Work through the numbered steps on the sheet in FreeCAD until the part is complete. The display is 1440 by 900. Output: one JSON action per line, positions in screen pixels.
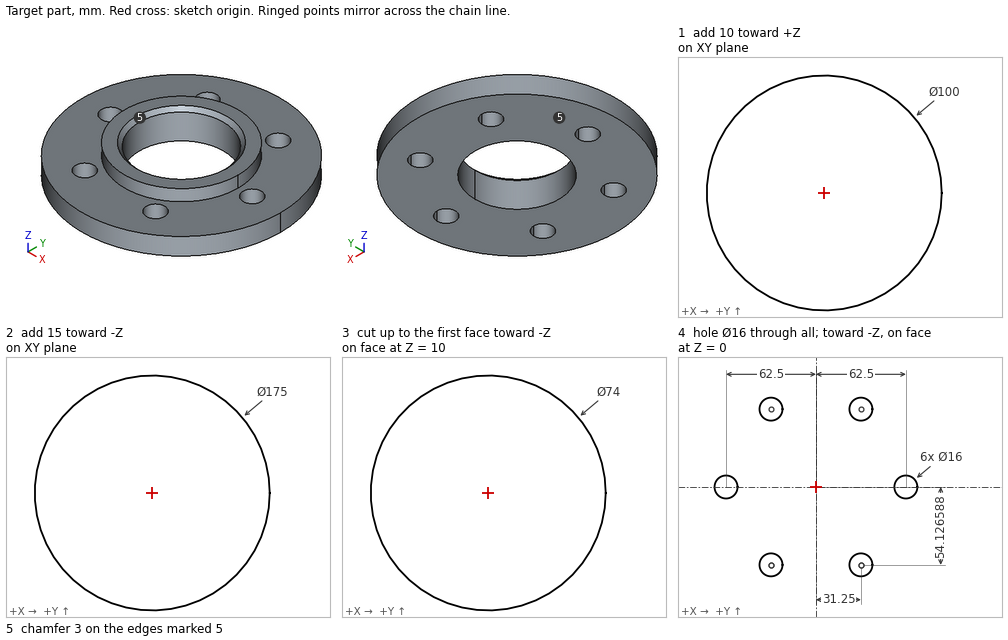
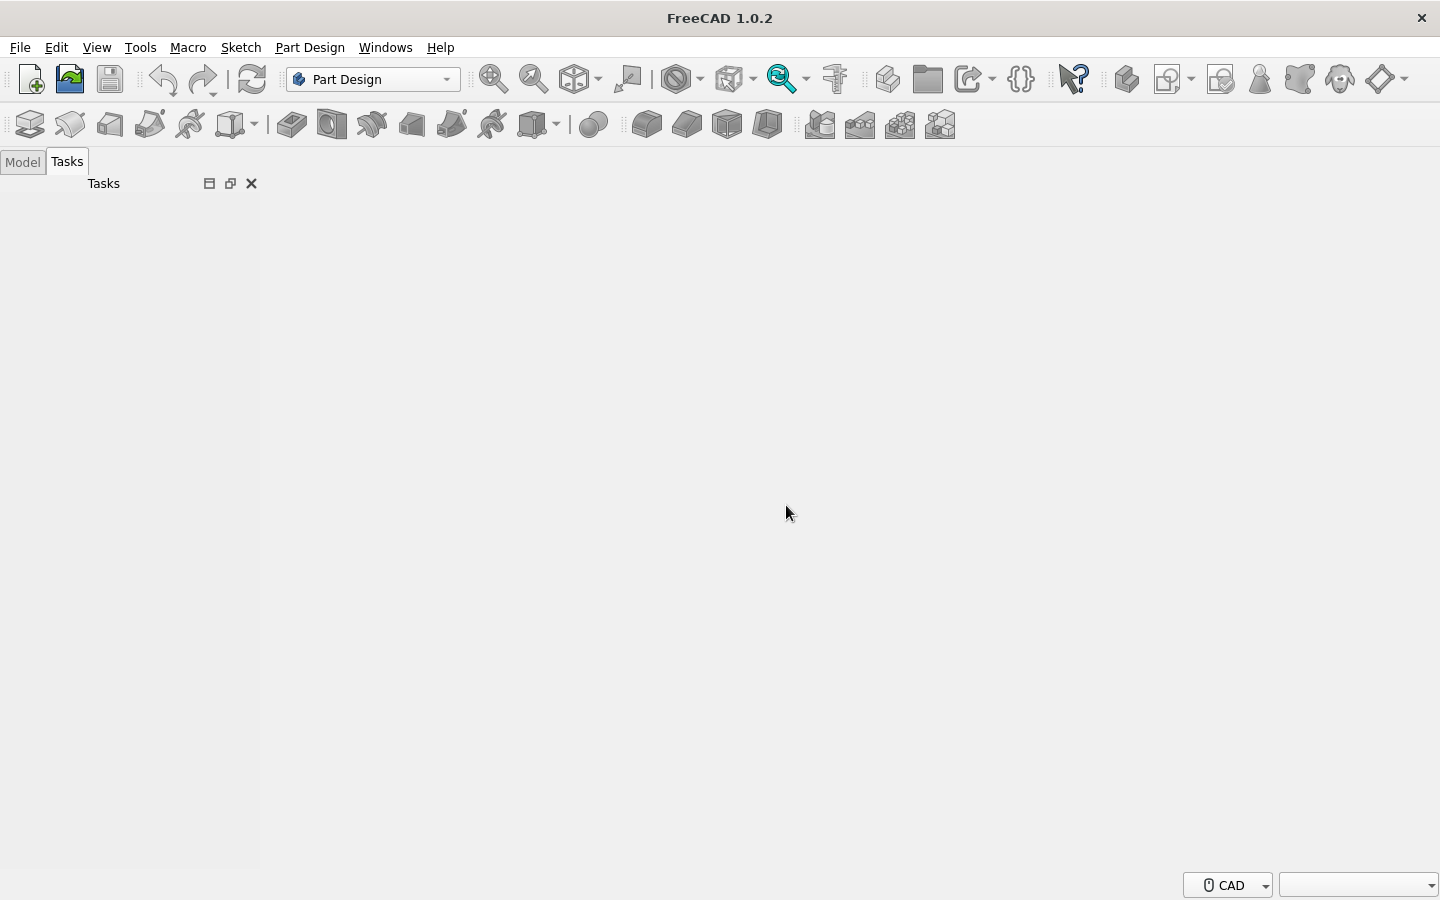
{"action": "left_click", "coordinate": [30, 80]}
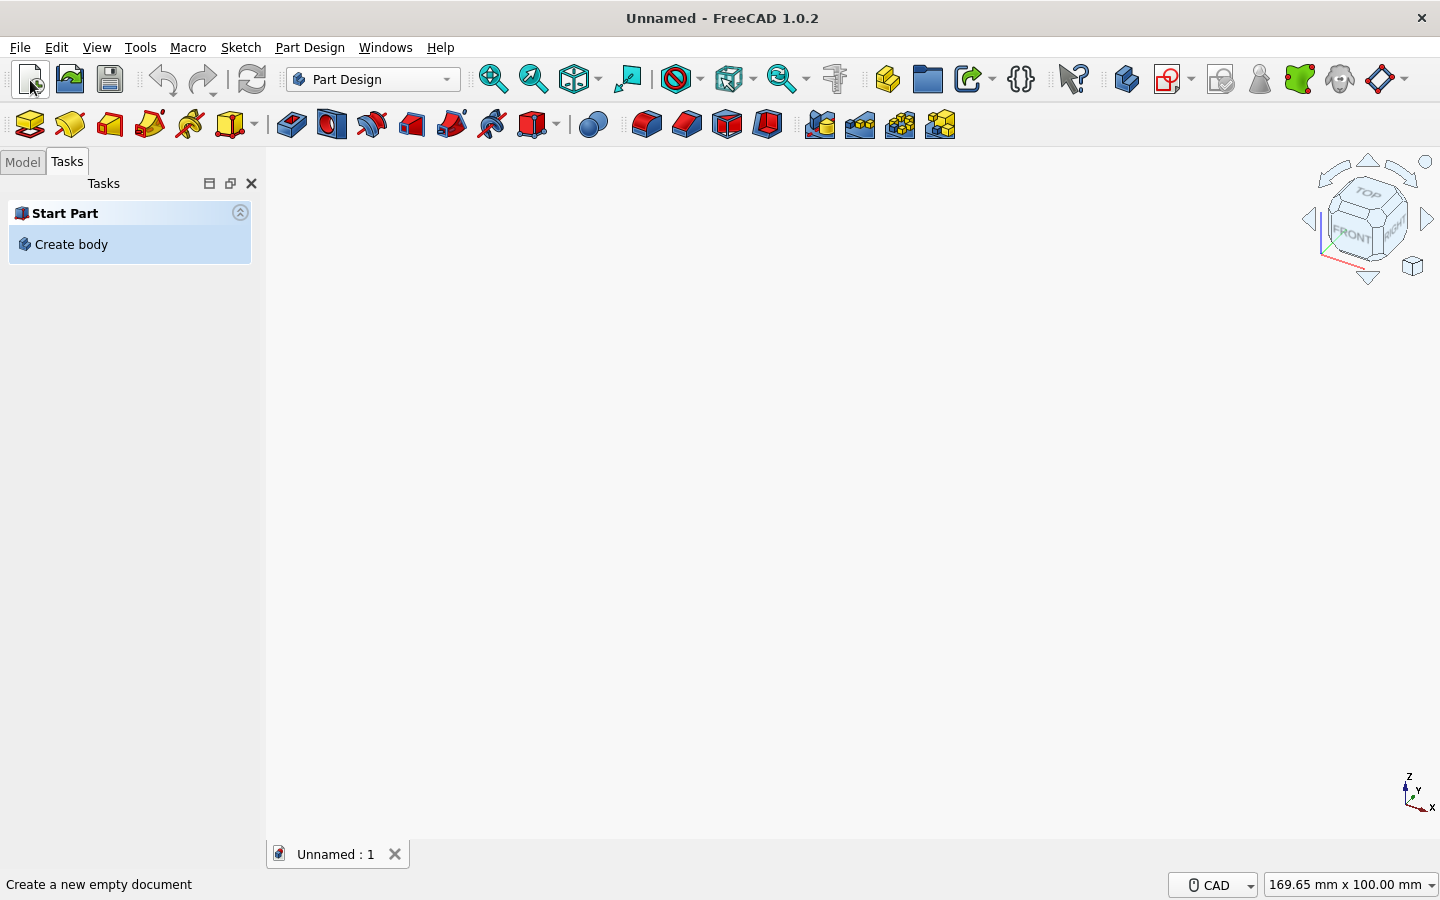
{"action": "left_click", "coordinate": [1168, 80]}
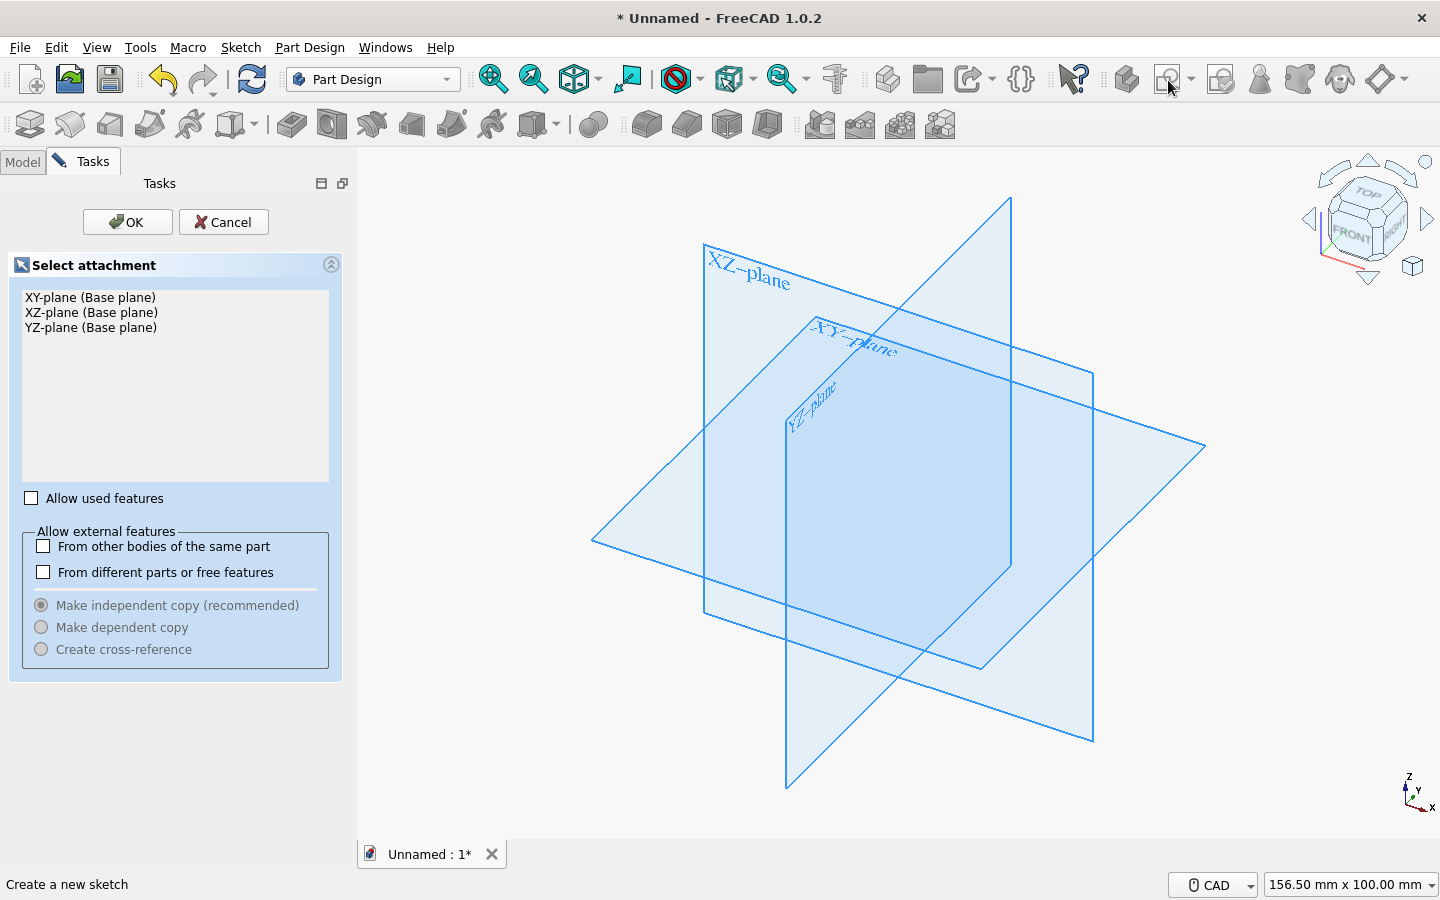
{"action": "left_click", "coordinate": [82, 298]}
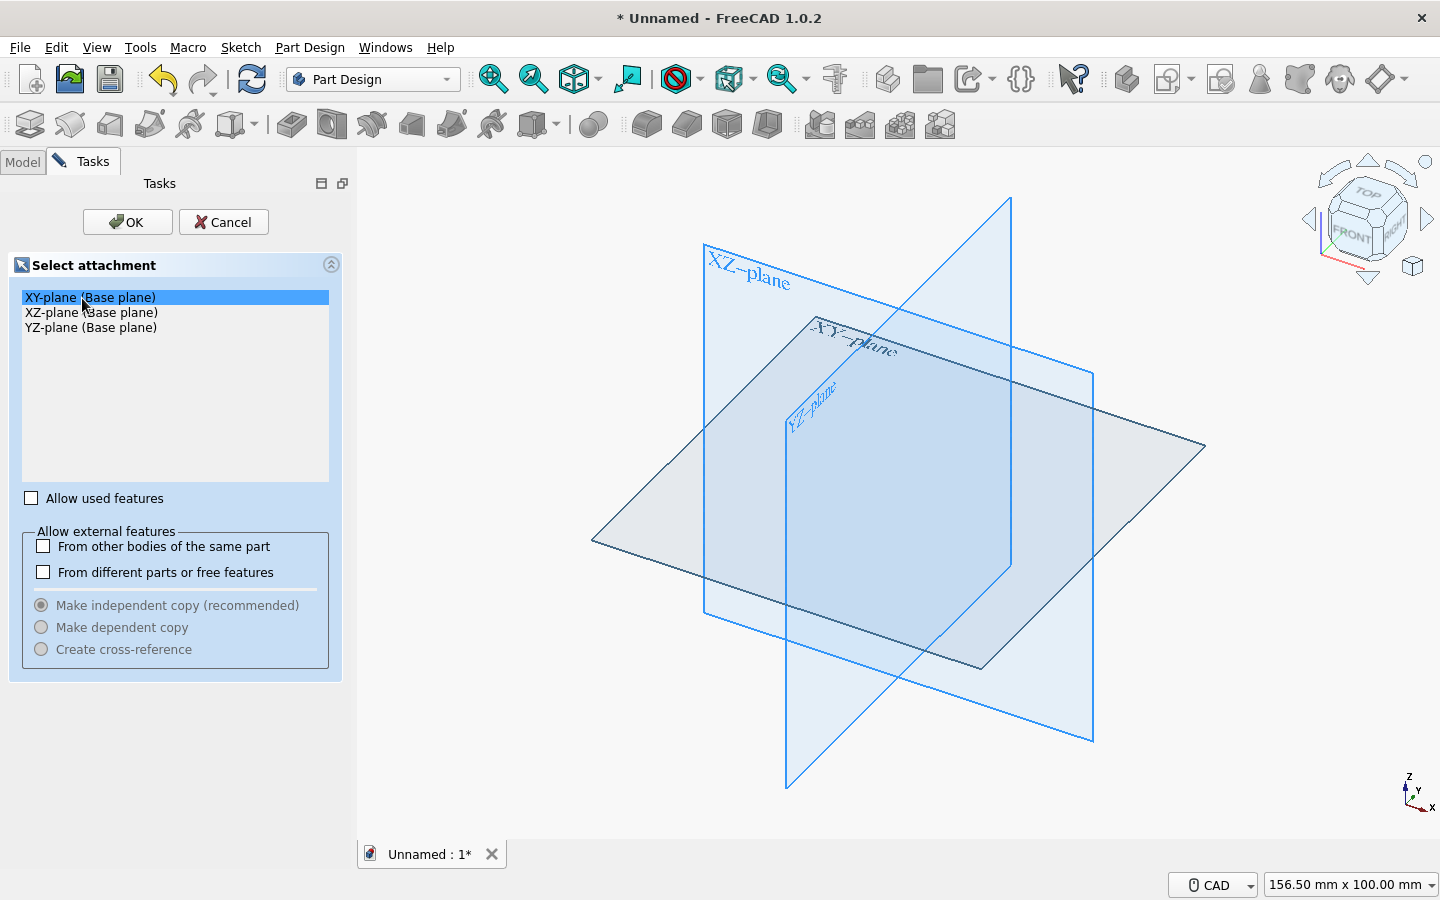
{"action": "left_click", "coordinate": [128, 222]}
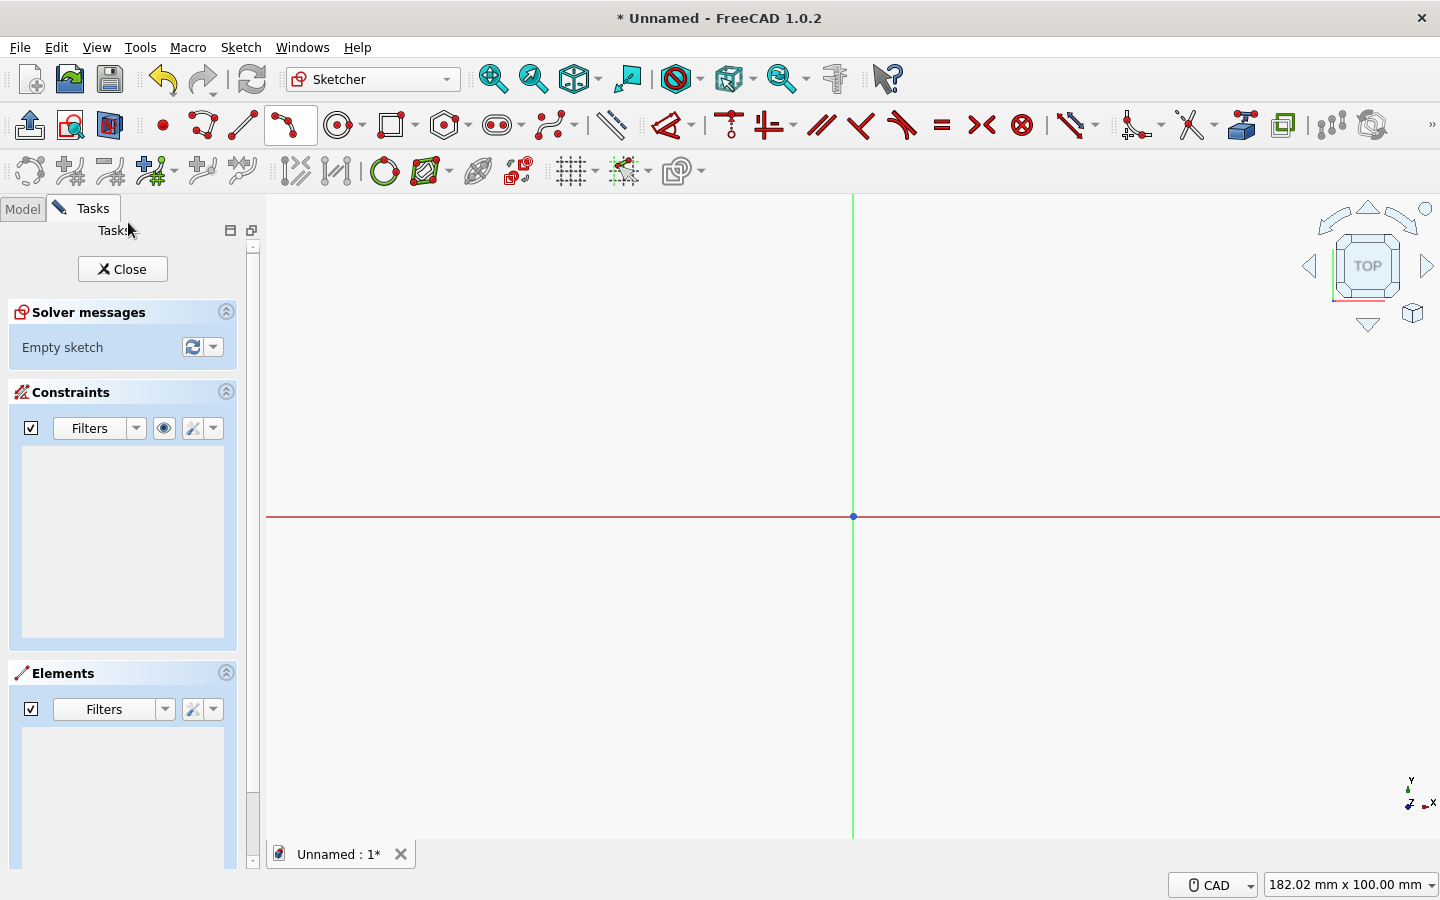
{"action": "scroll", "coordinate": [645, 516], "scroll_direction": "down", "scroll_amount": 2}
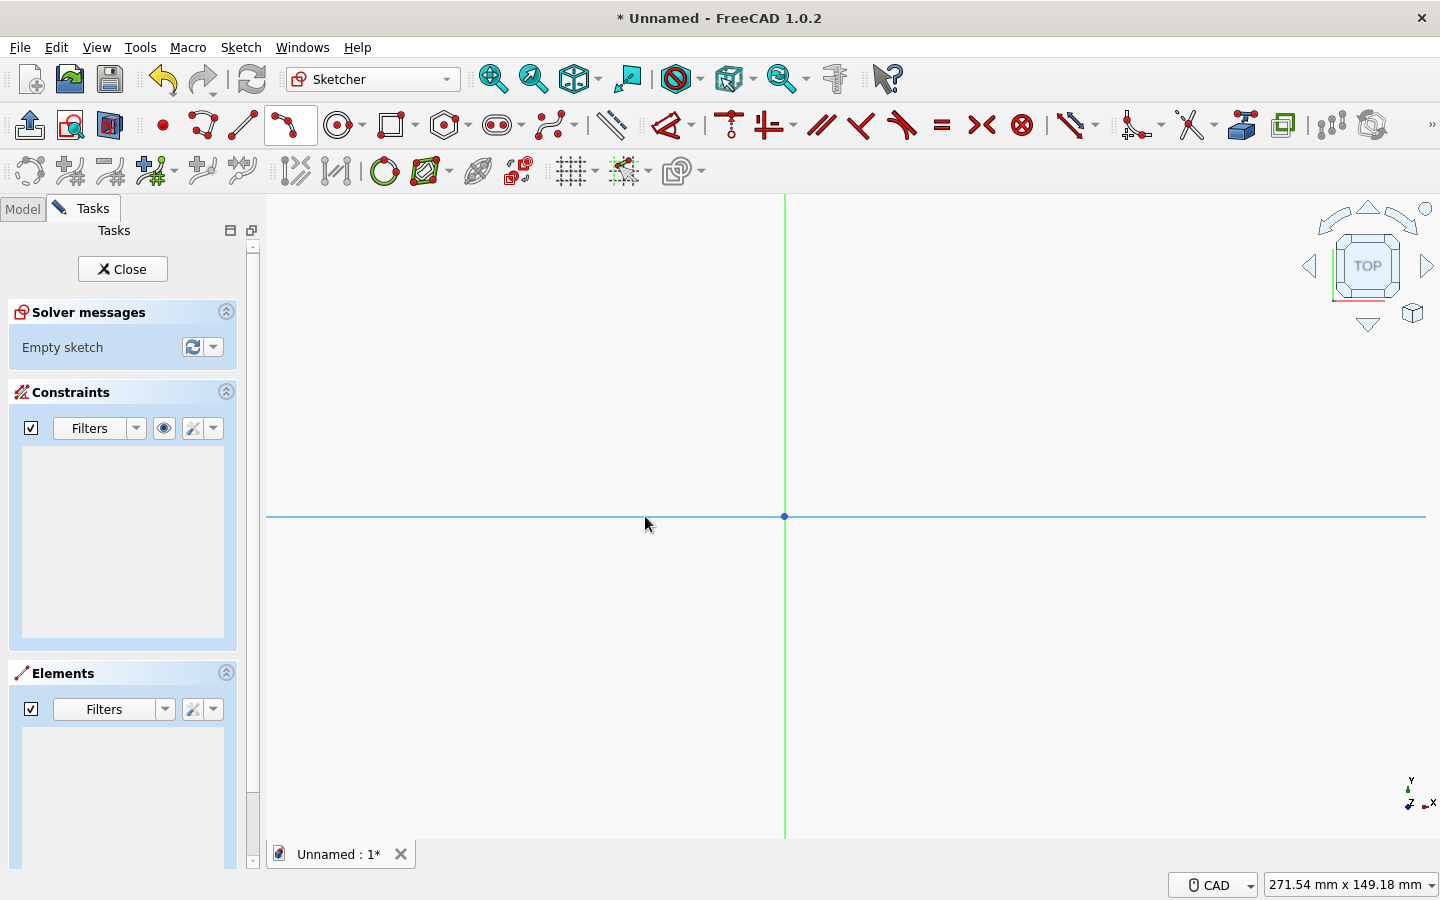
{"action": "left_click", "coordinate": [338, 126]}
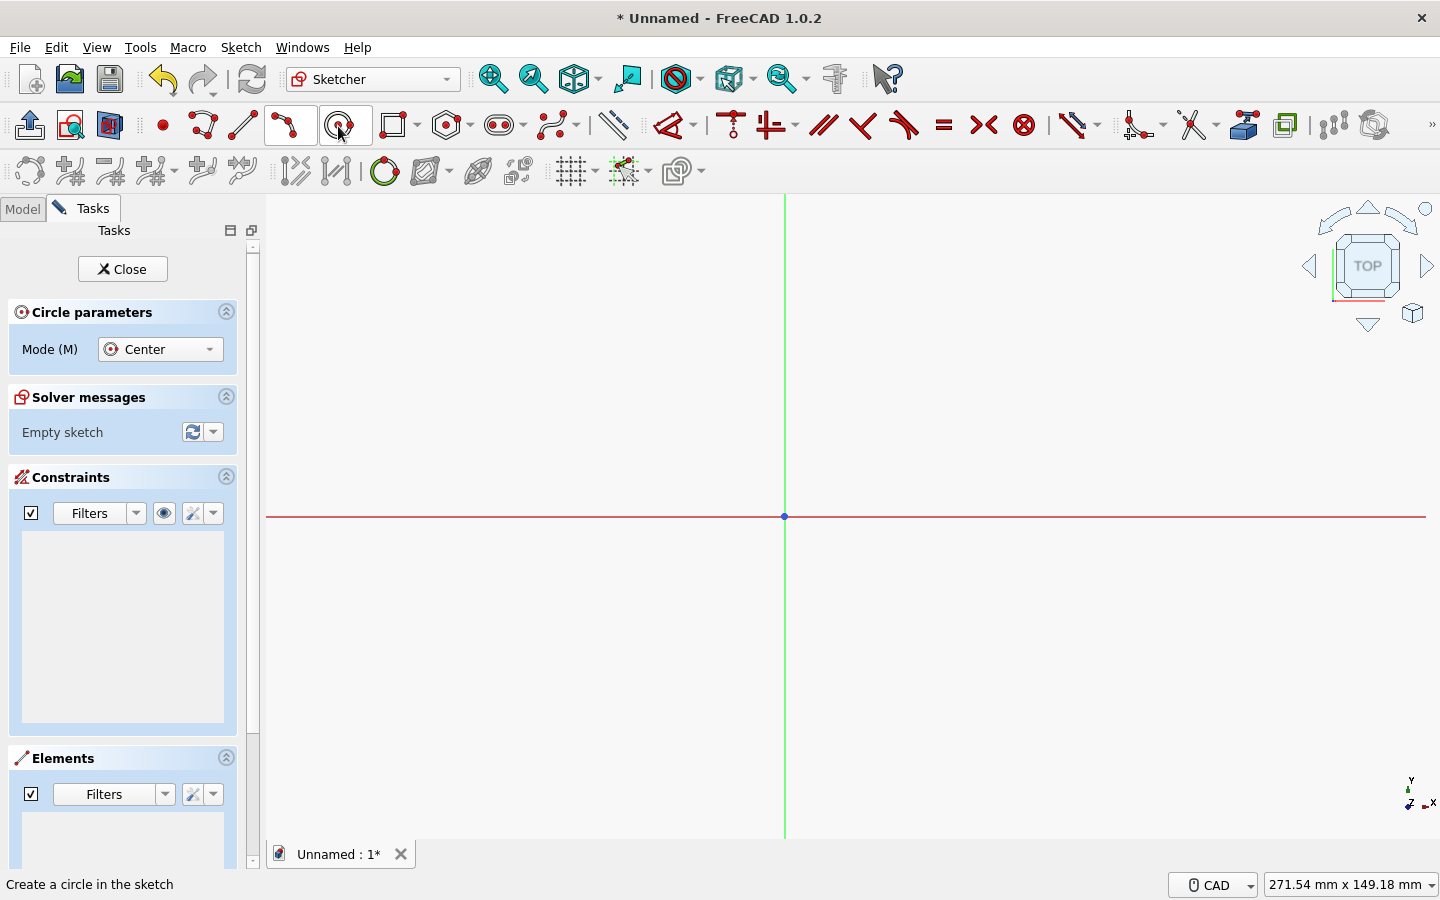
{"action": "left_click", "coordinate": [785, 516]}
{"action": "left_click", "coordinate": [937, 364]}
{"action": "key", "text": "Escape"}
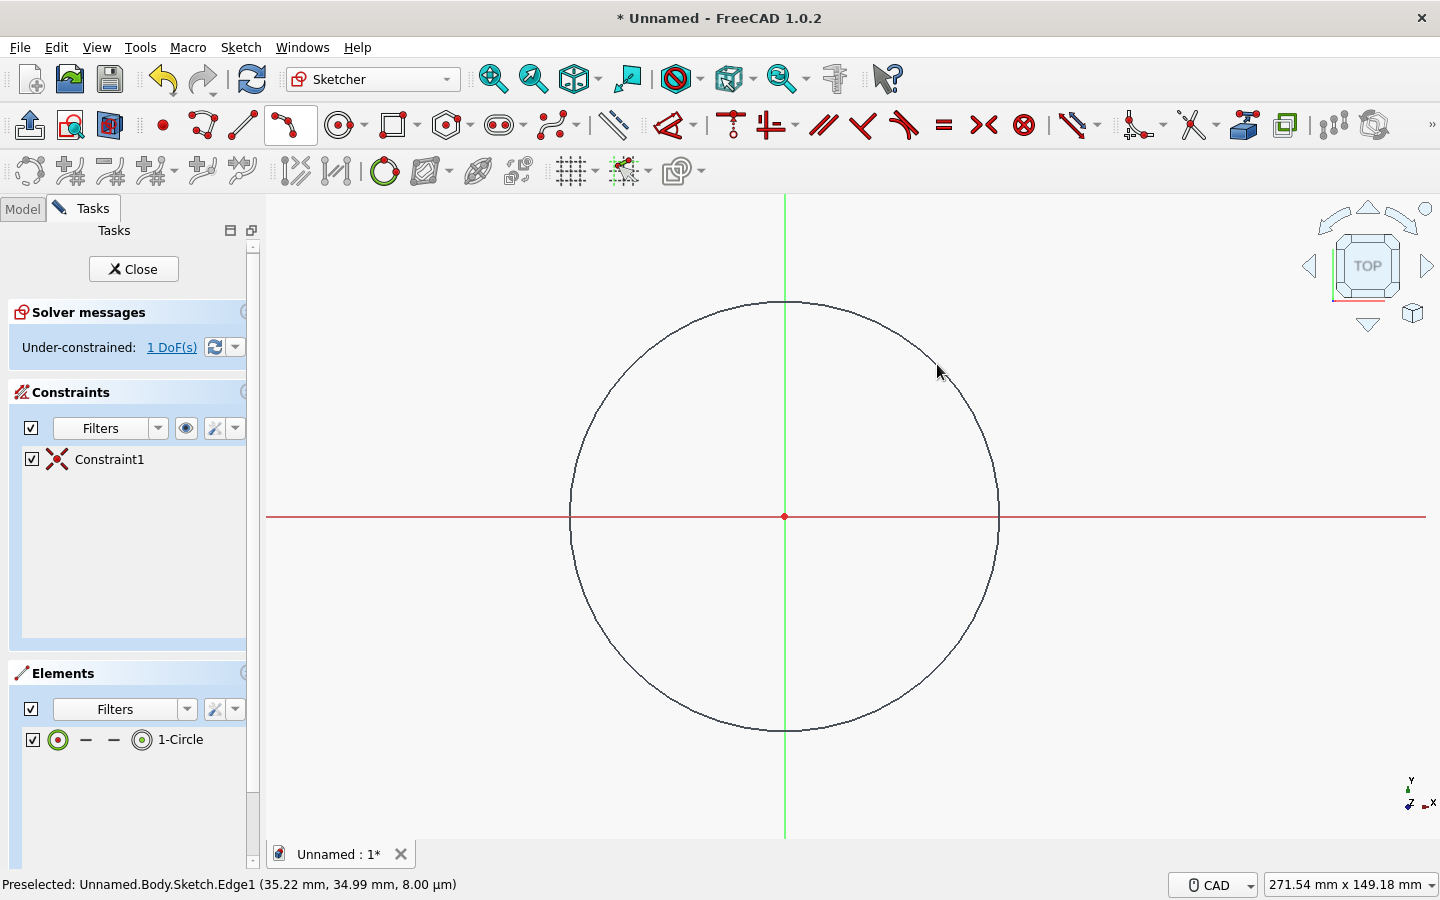
{"action": "left_click", "coordinate": [668, 126]}